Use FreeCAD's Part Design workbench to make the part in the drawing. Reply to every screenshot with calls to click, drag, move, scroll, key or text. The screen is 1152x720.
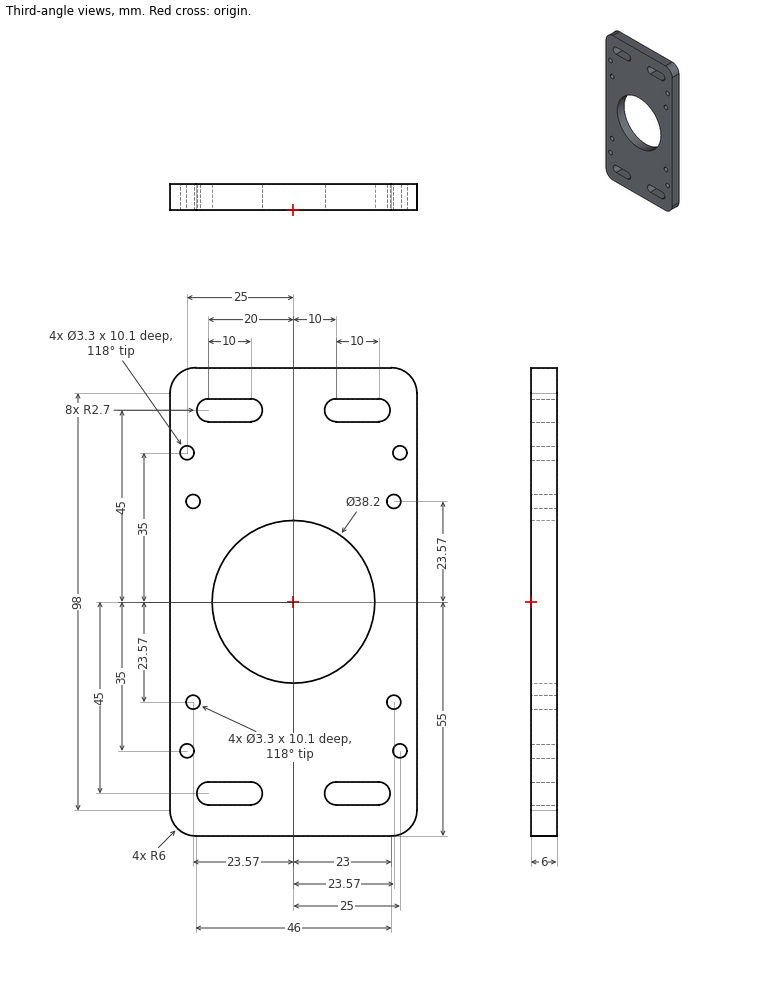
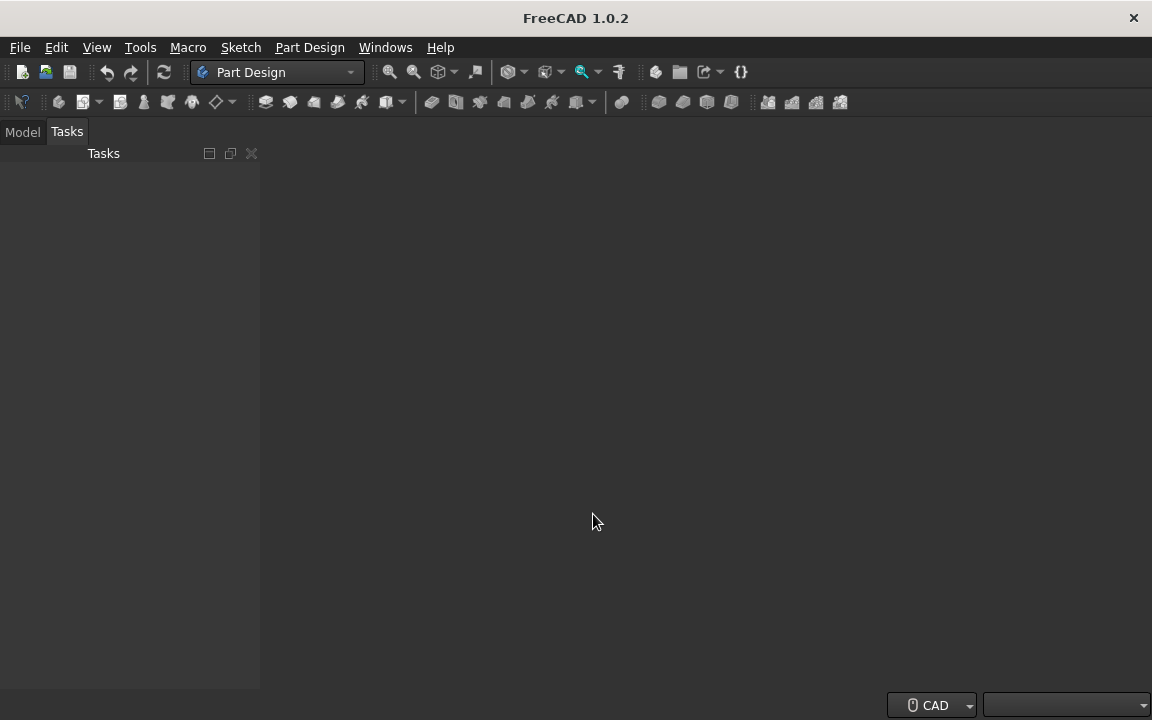
click(22, 72)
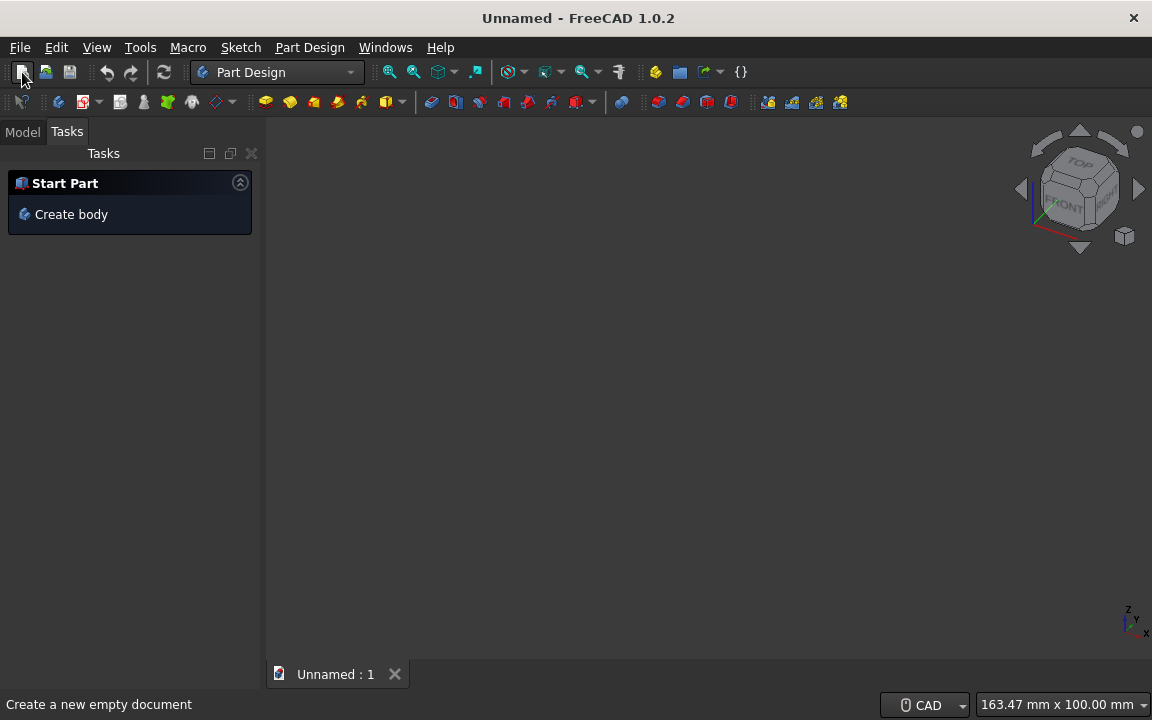
click(84, 102)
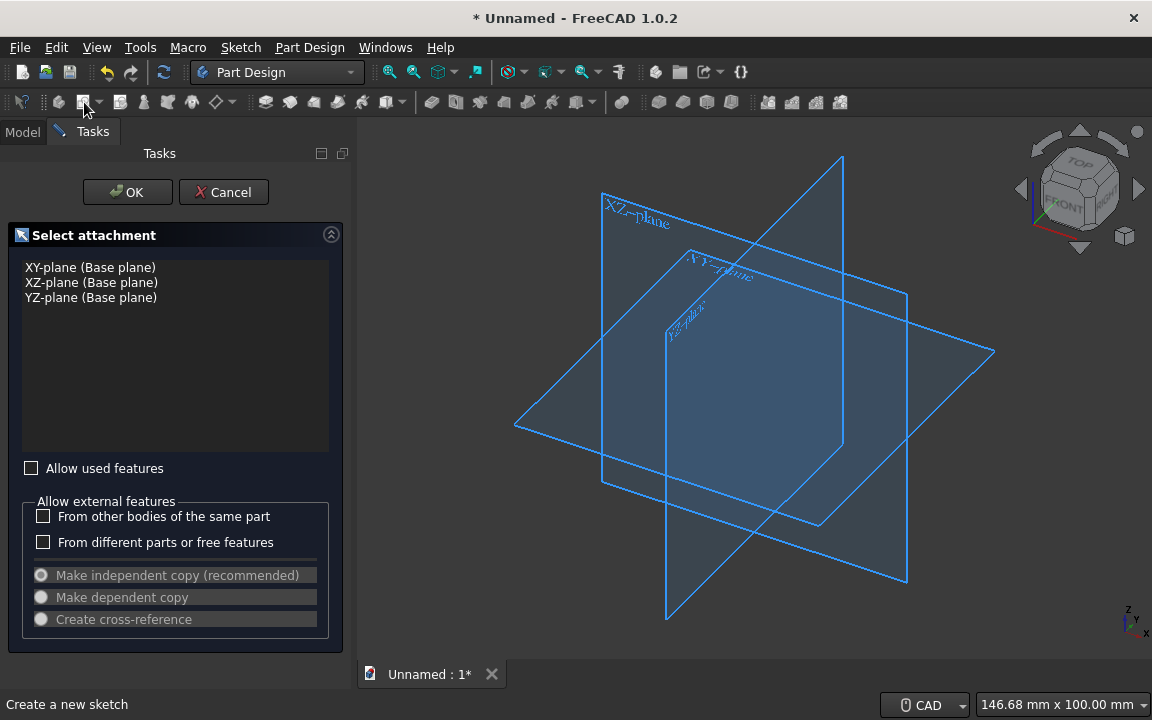
click(82, 282)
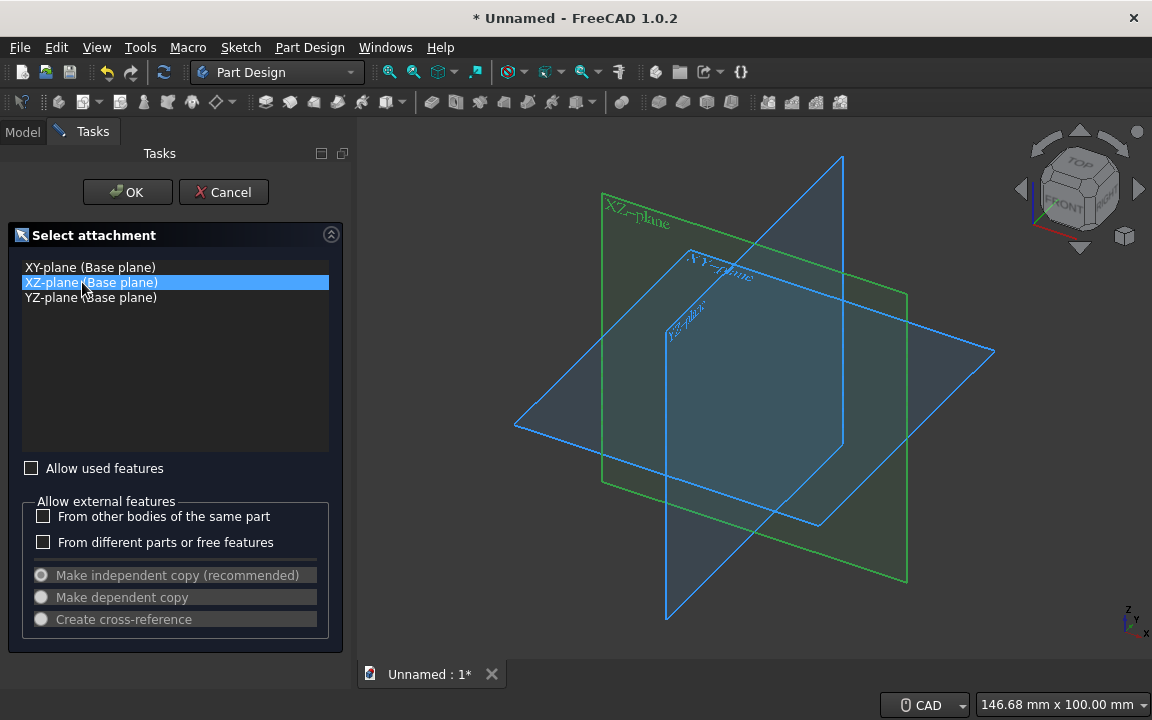
click(128, 192)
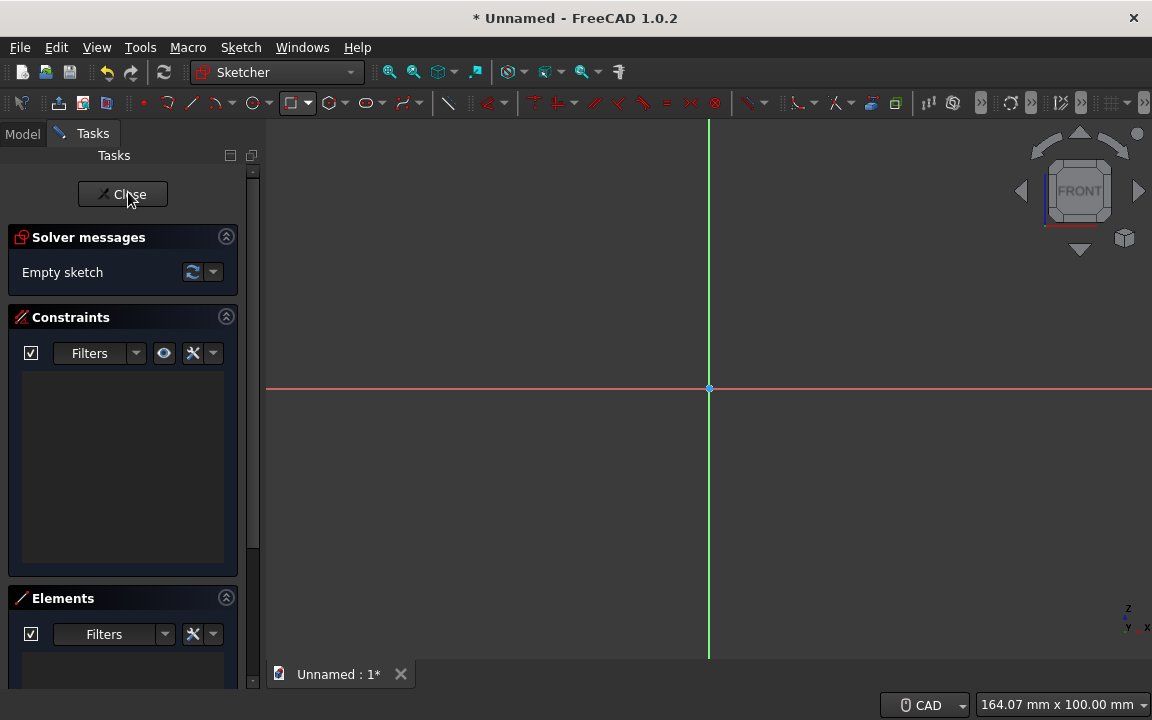
scroll(557, 389, down, 3)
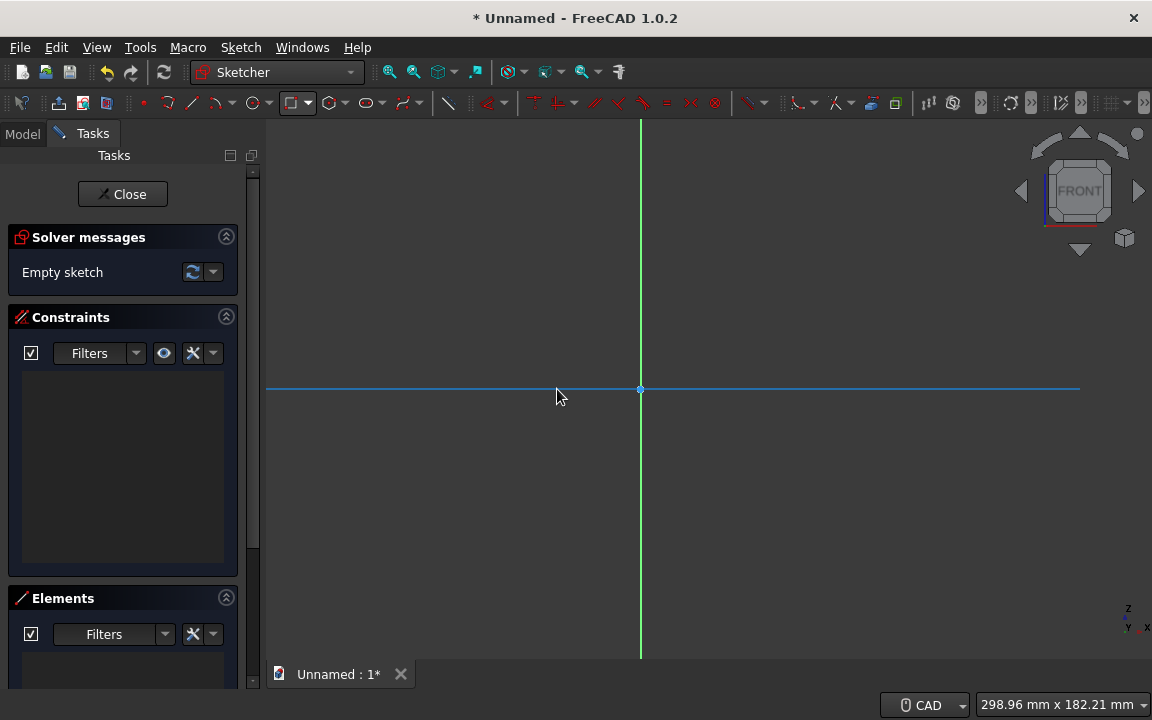
click(192, 104)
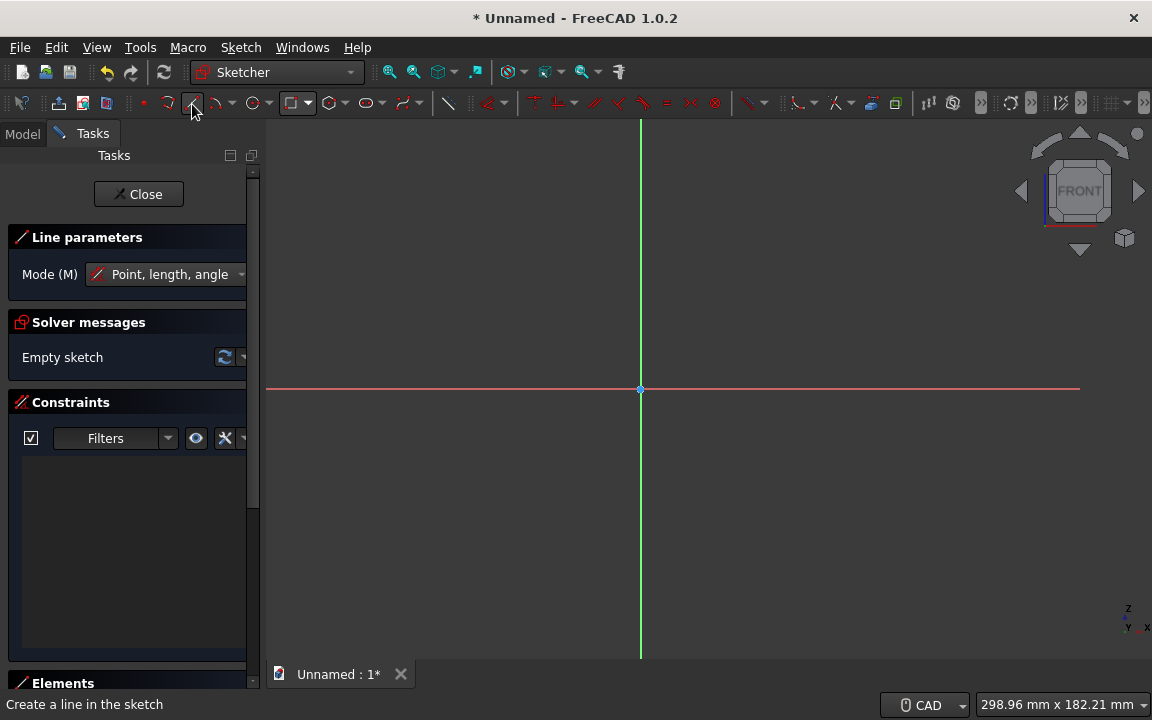
click(709, 552)
click(572, 552)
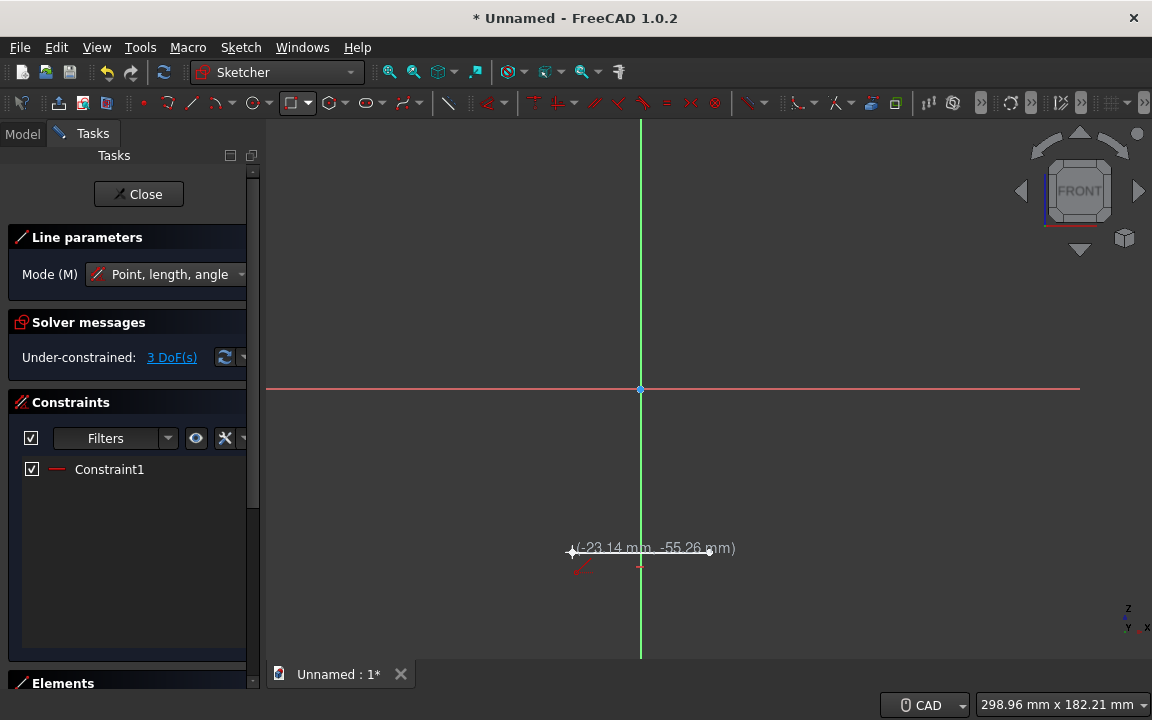
click(555, 534)
click(555, 244)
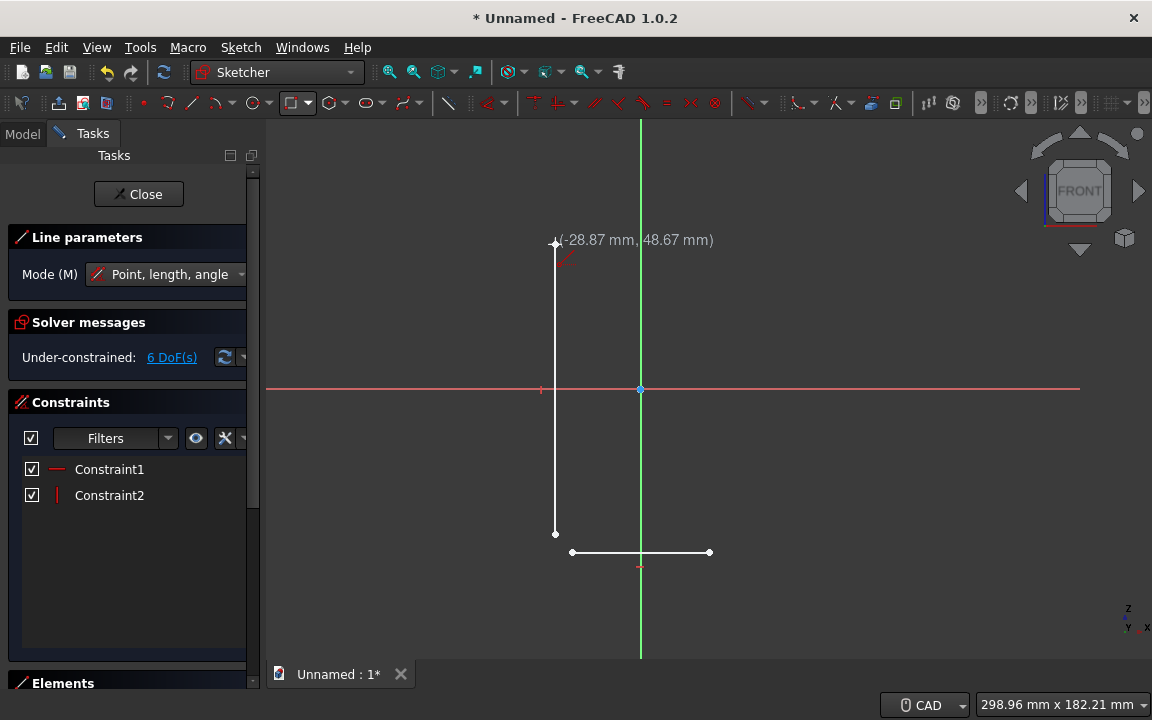
click(572, 226)
click(709, 226)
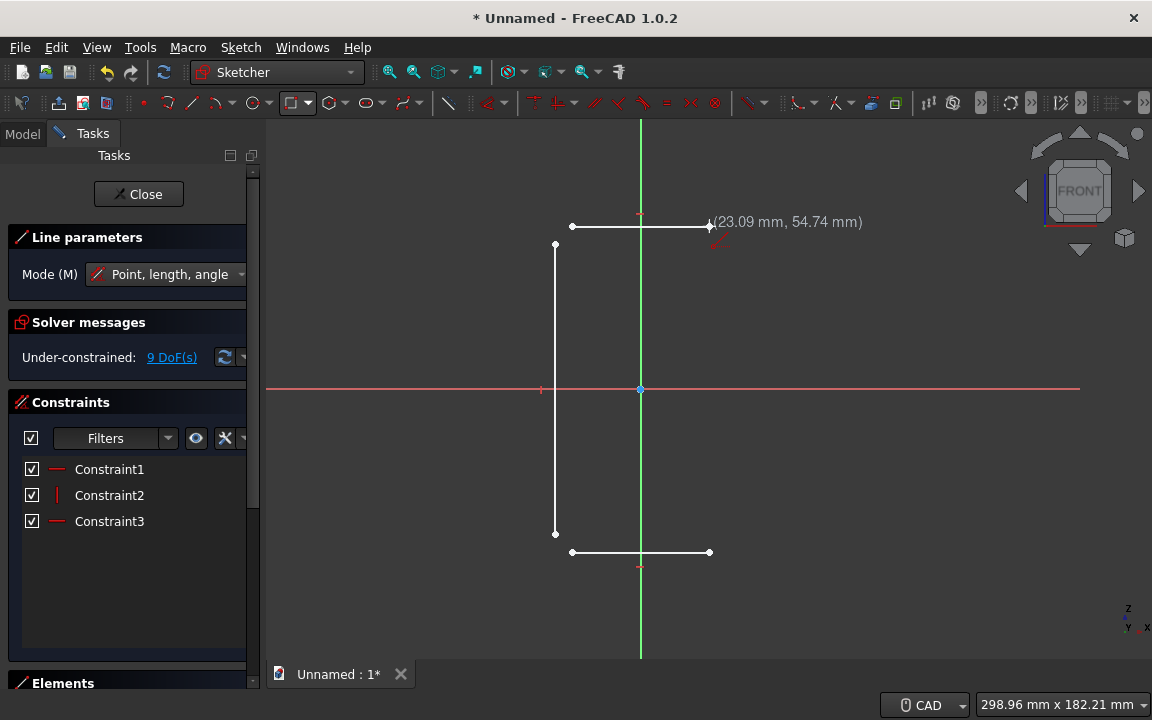
click(727, 244)
click(727, 534)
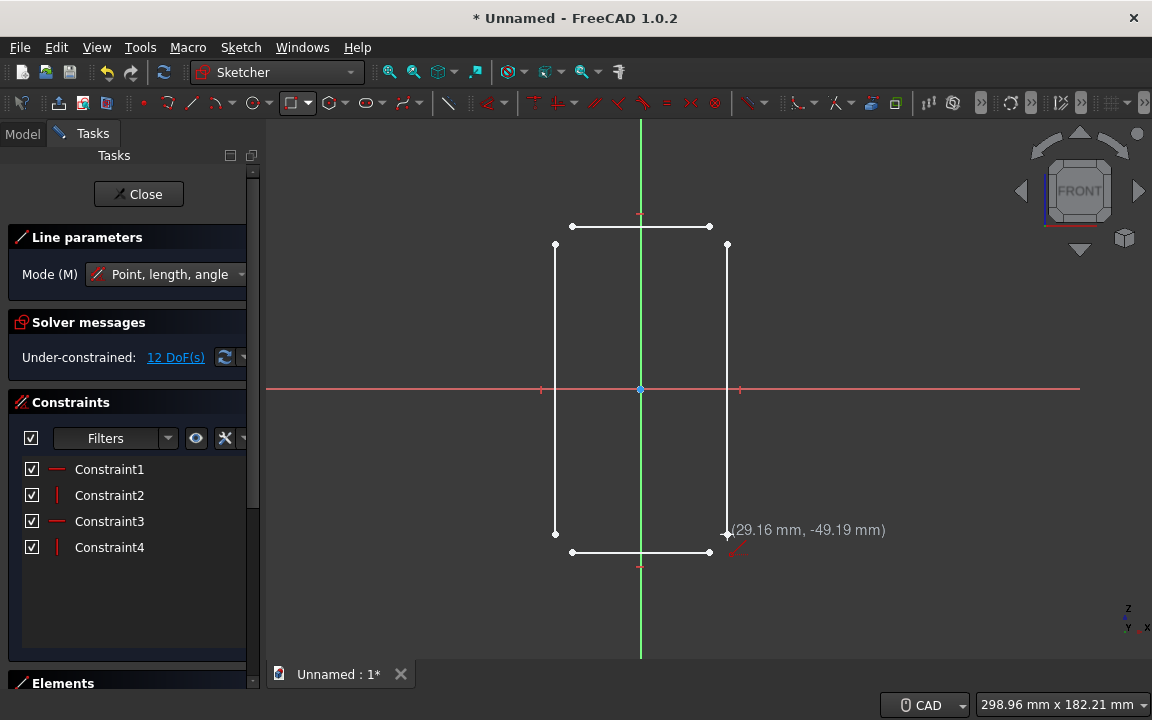
click(234, 104)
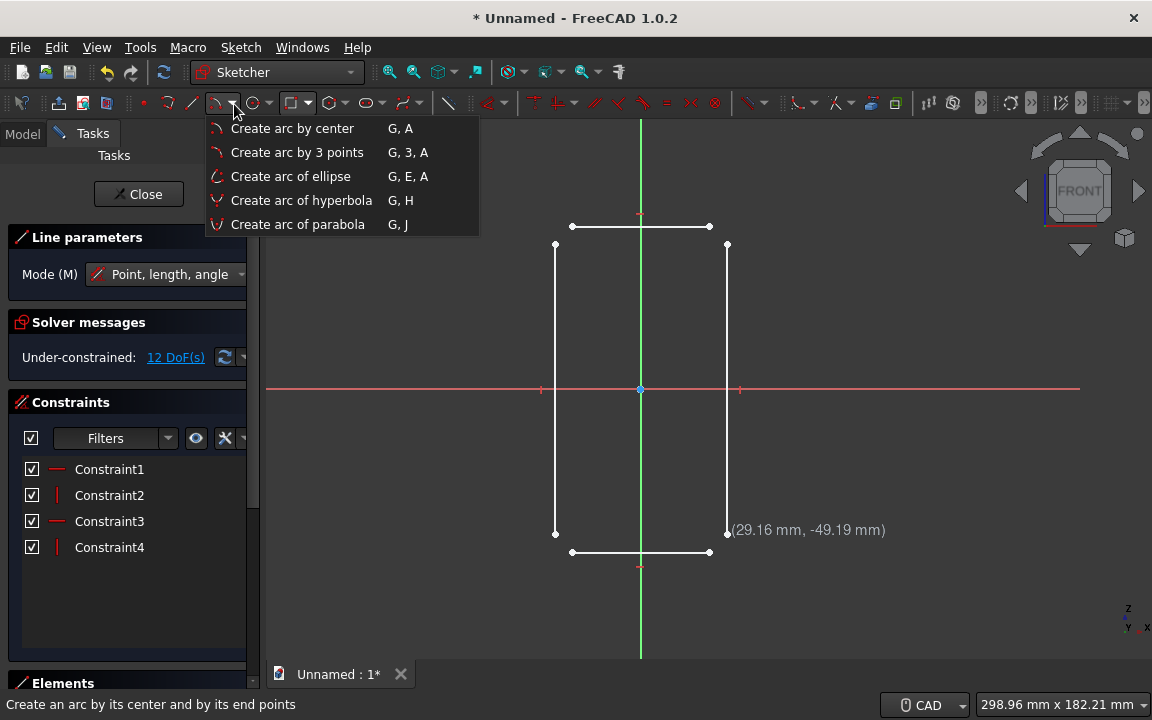
click(342, 152)